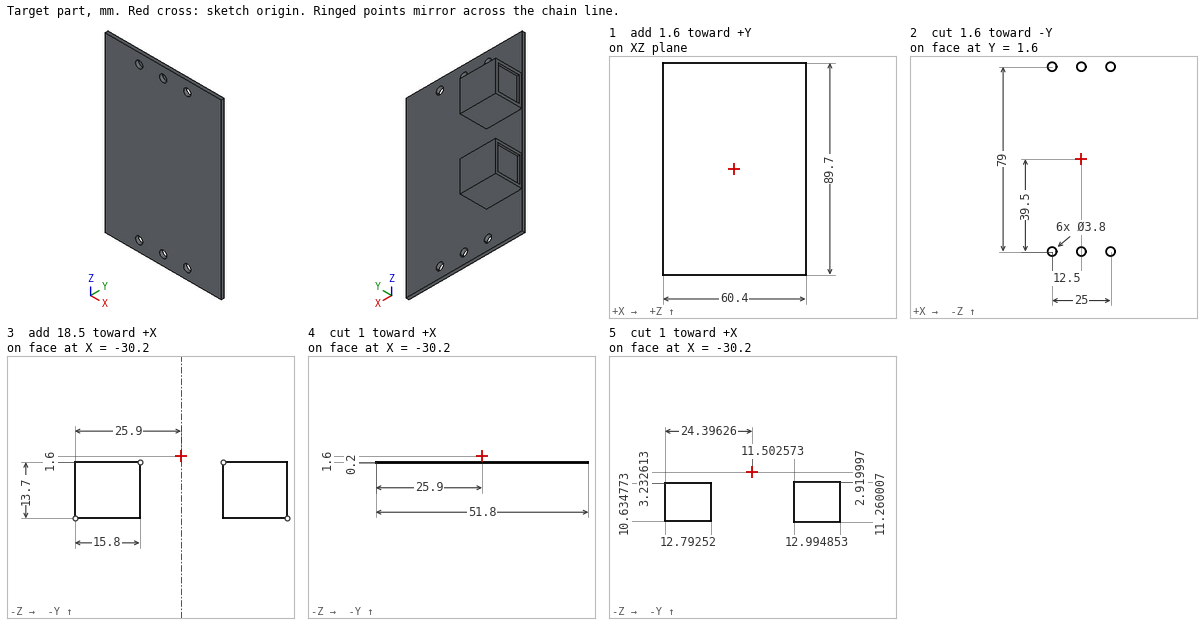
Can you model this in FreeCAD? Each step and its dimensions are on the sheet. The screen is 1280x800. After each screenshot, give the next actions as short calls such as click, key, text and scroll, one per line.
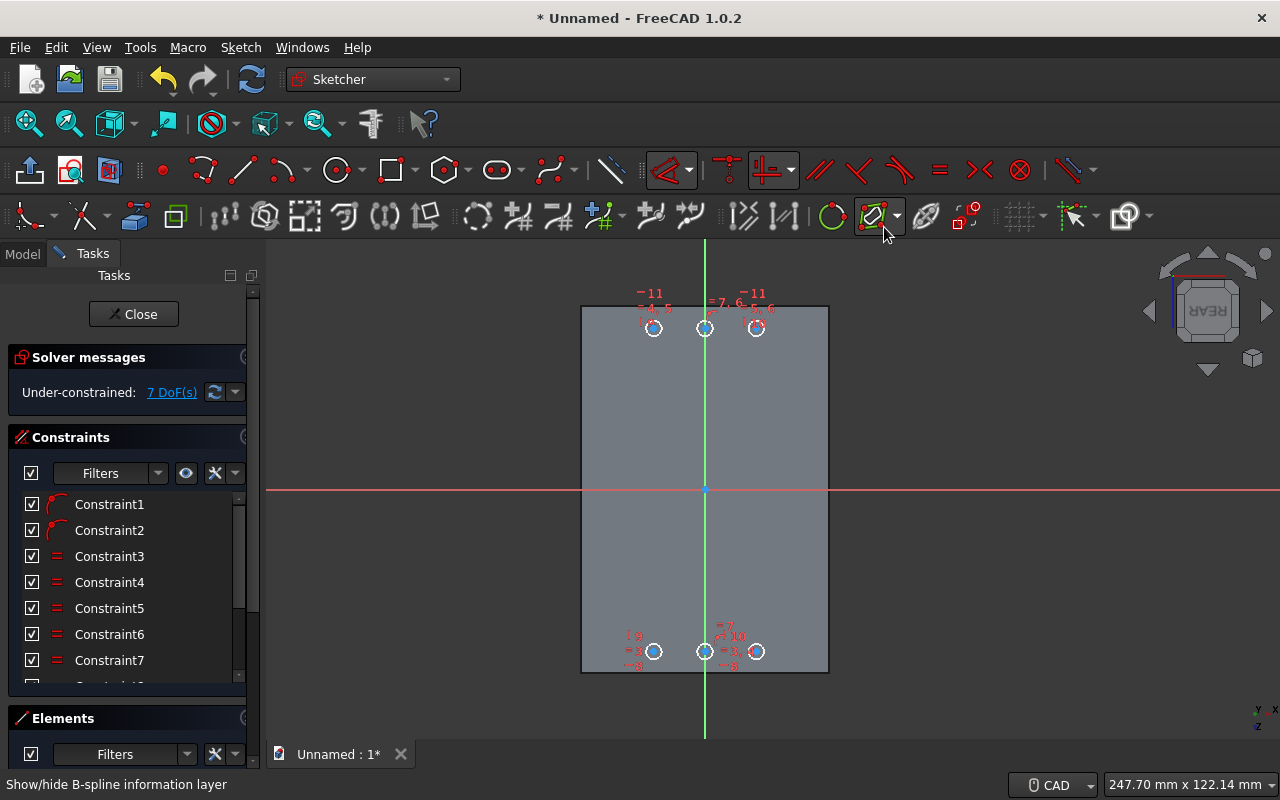
click(654, 328)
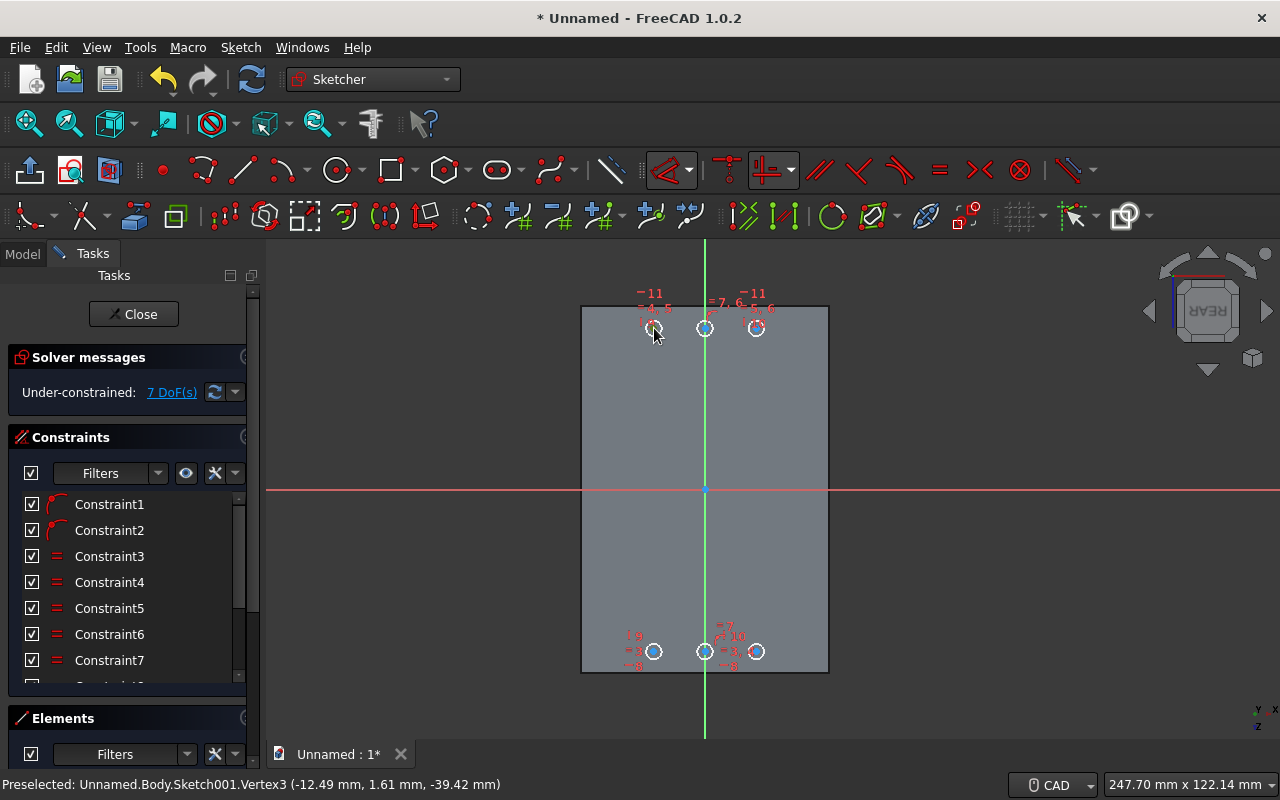
click(705, 328)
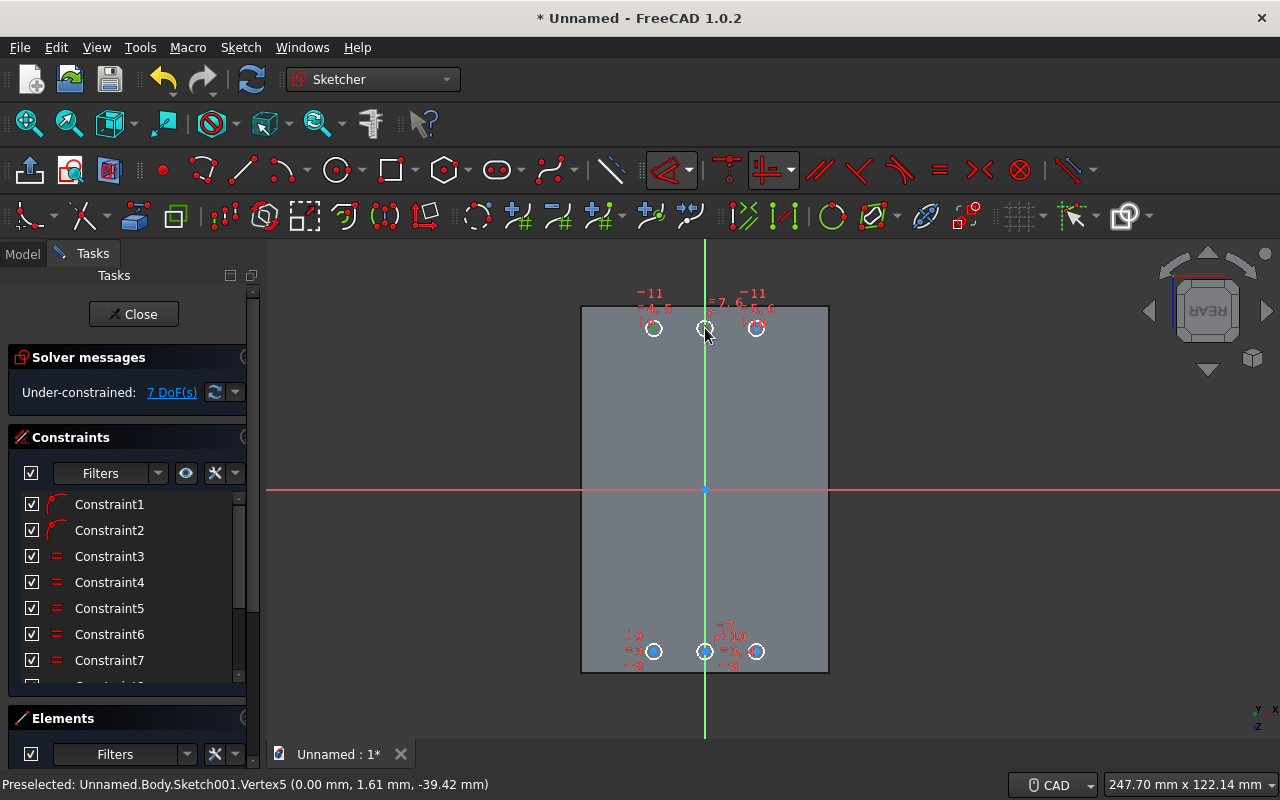
key(h)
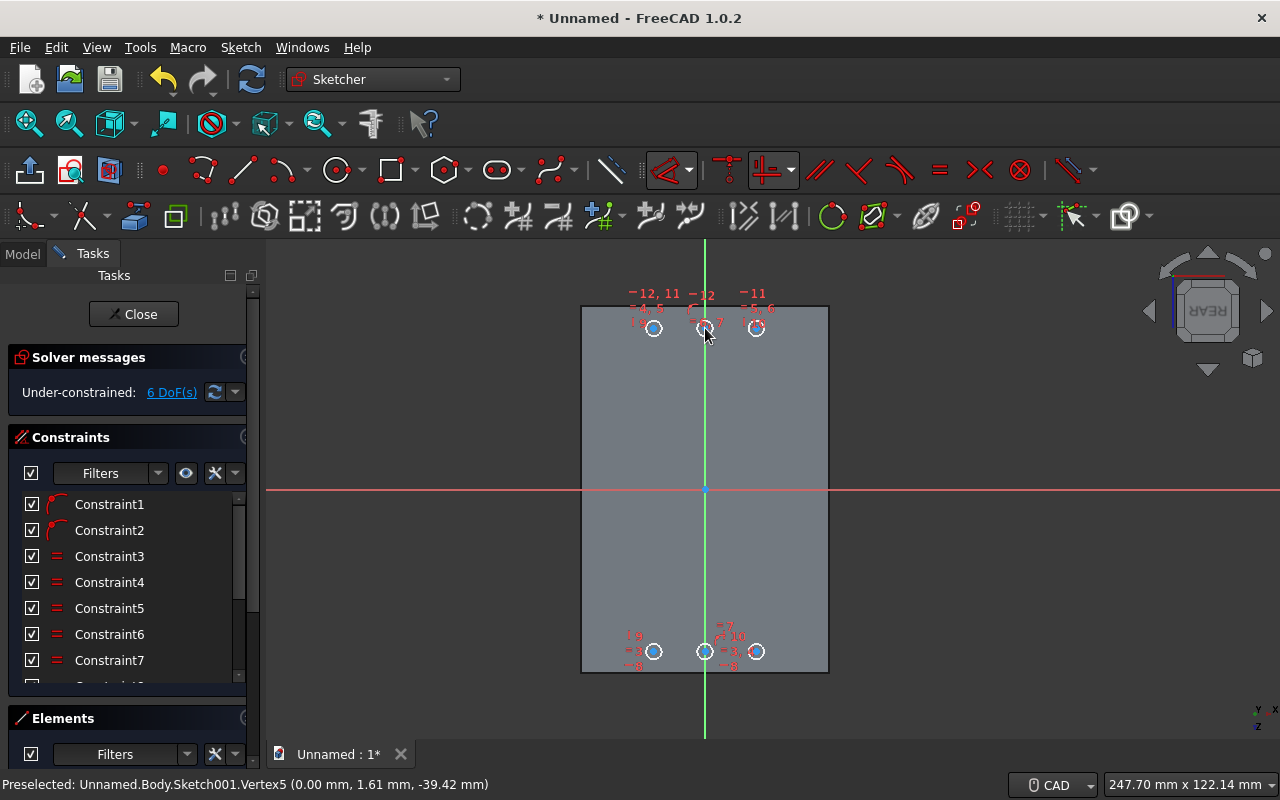
click(654, 652)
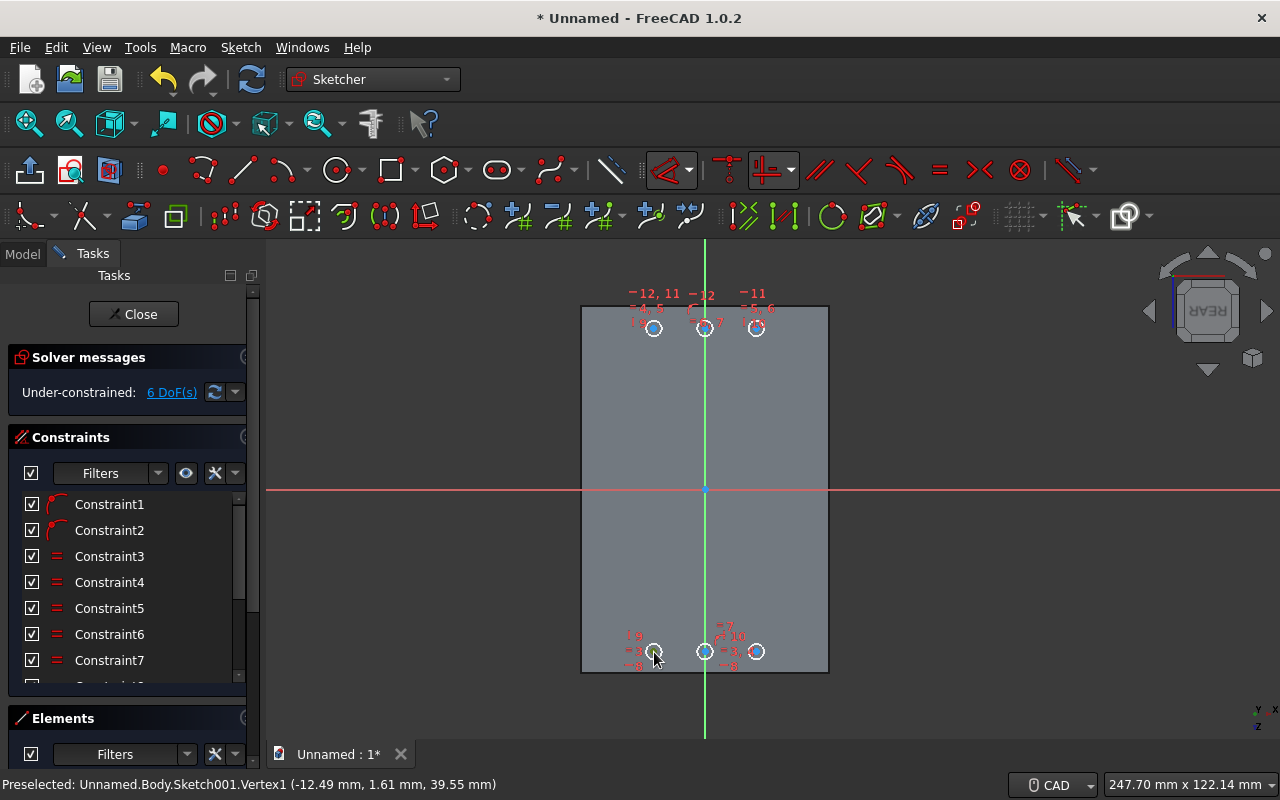
click(705, 652)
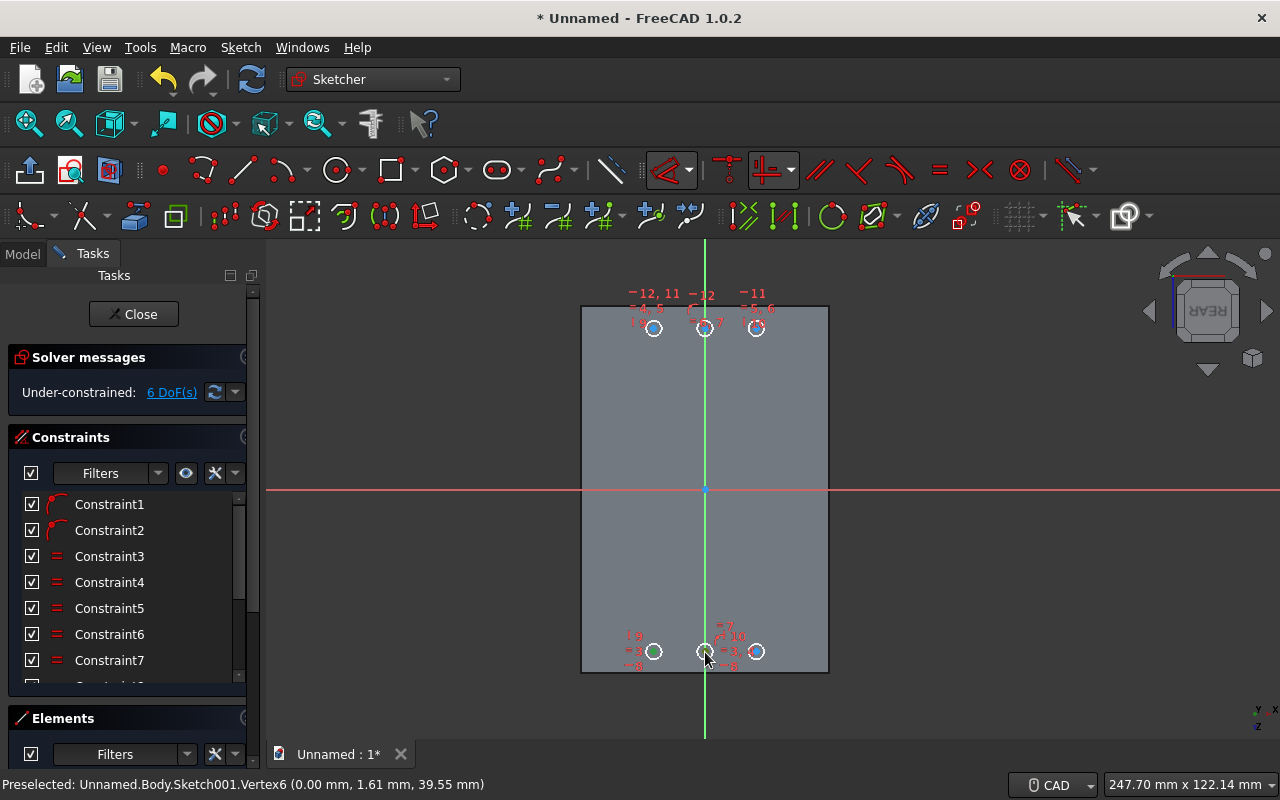
key(h)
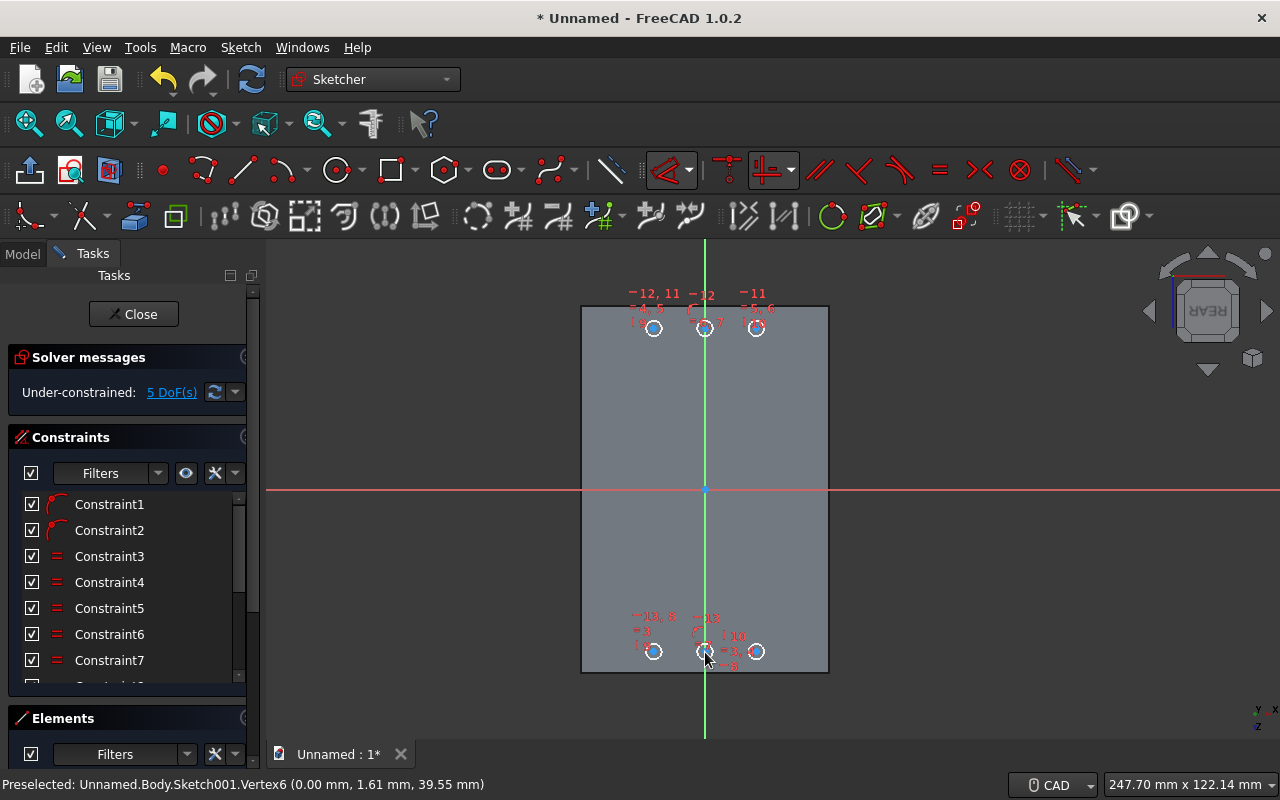
click(666, 170)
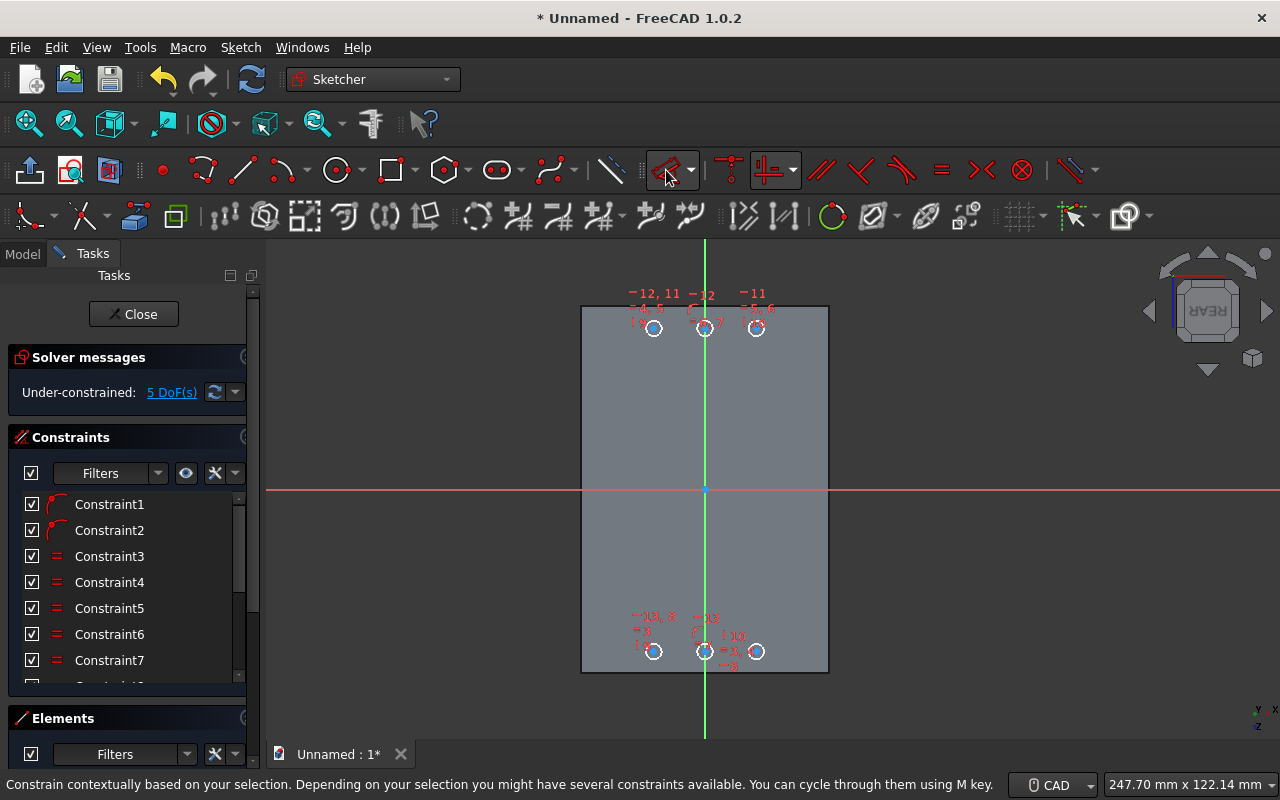
scroll(659, 646, up, 5)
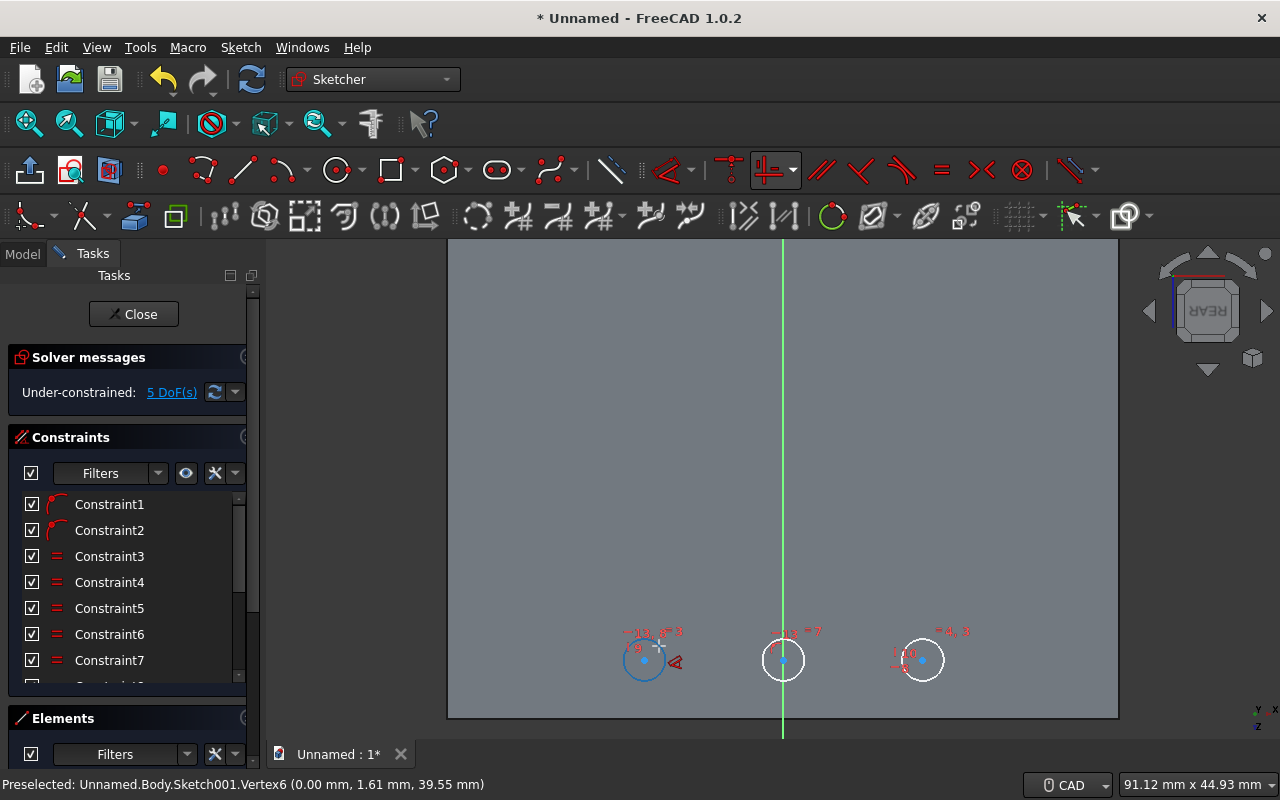
click(659, 645)
click(681, 622)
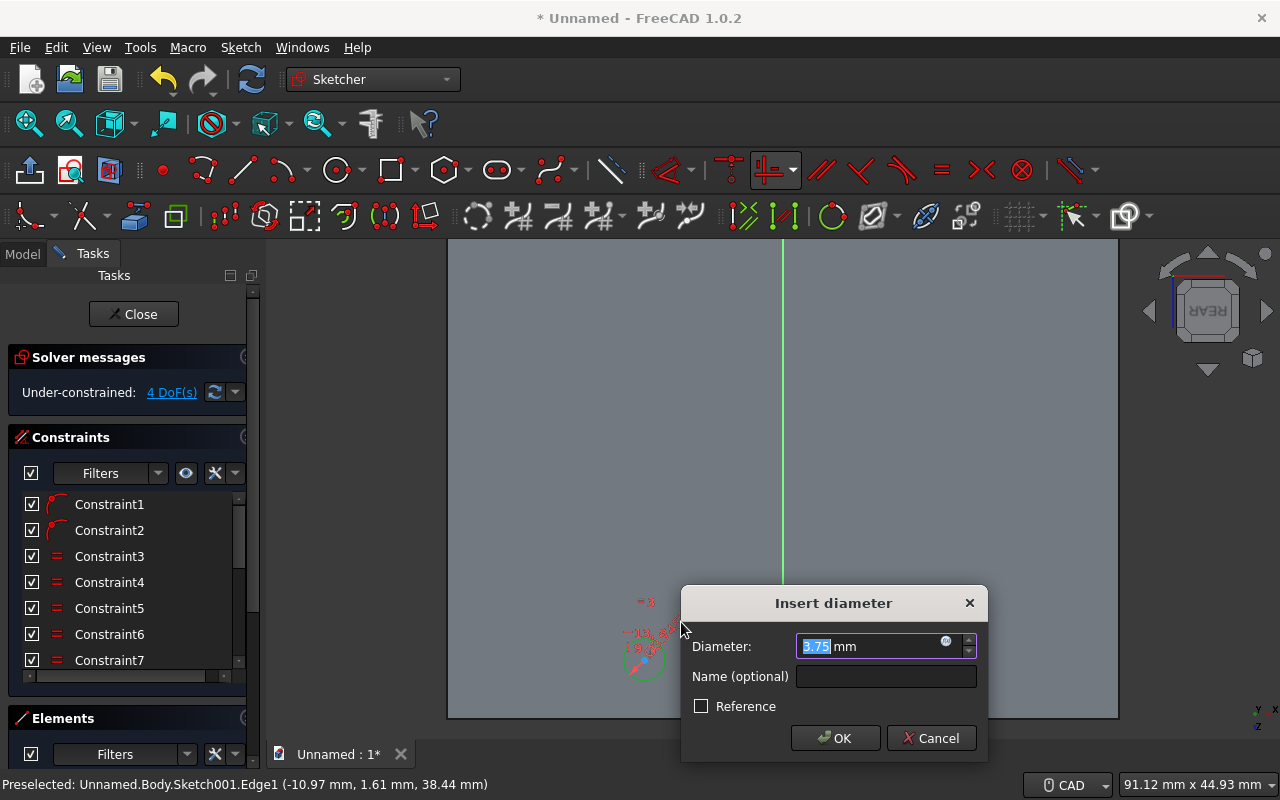
text(3.8)
key(Return)